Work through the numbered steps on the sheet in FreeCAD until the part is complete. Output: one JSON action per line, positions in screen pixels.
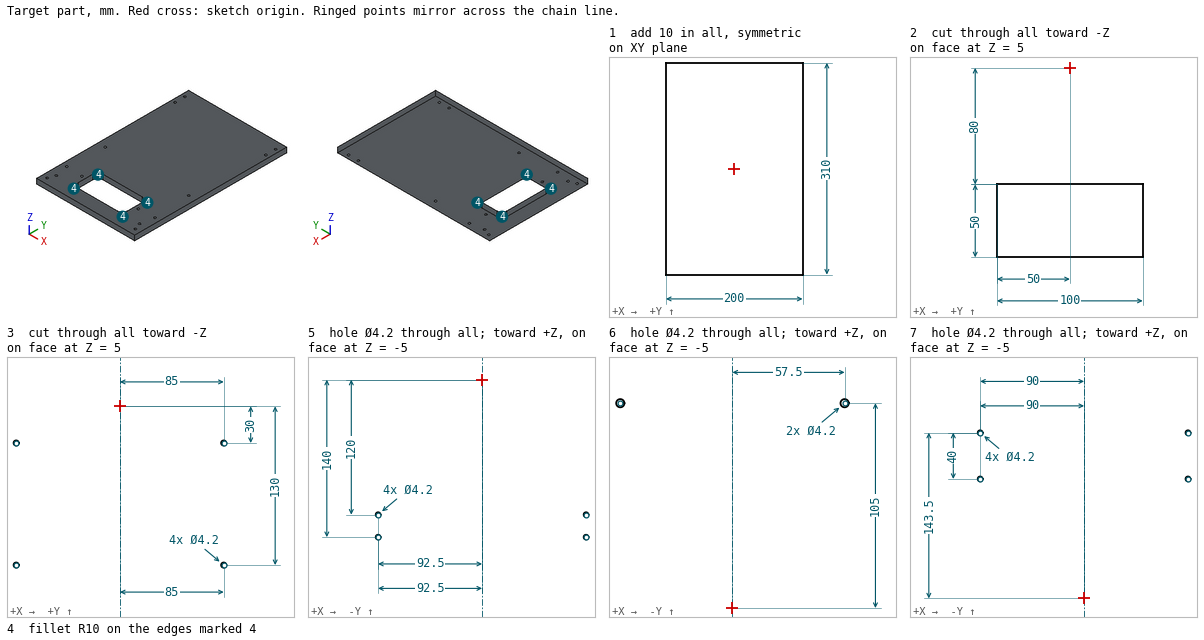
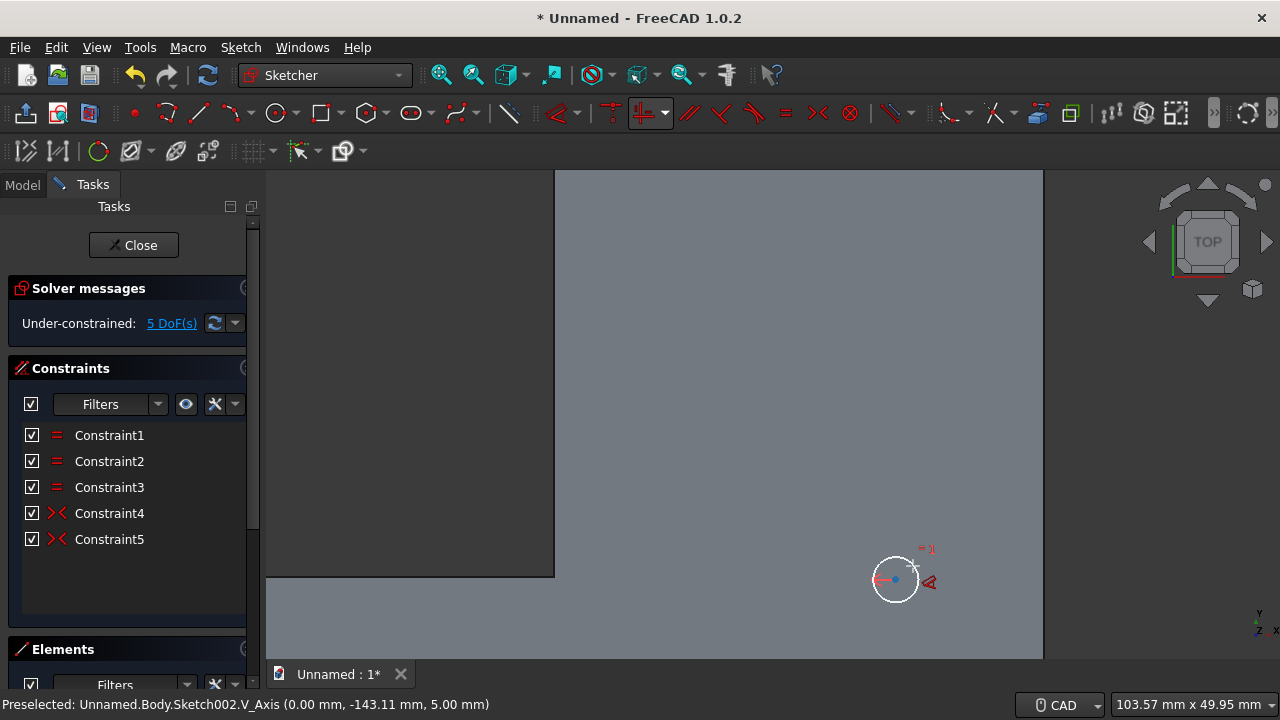
{"action": "left_click", "coordinate": [912, 564]}
{"action": "left_click", "coordinate": [935, 542]}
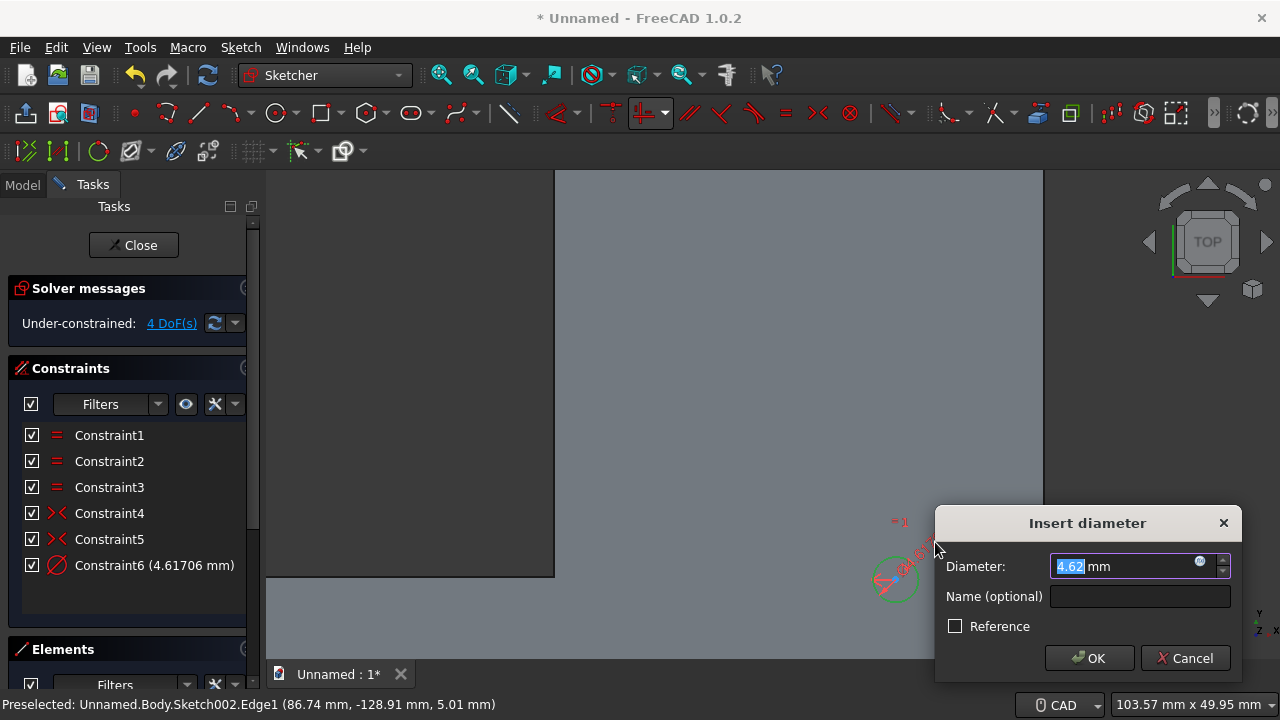
{"action": "type", "text": "4.2"}
{"action": "key", "text": "Return"}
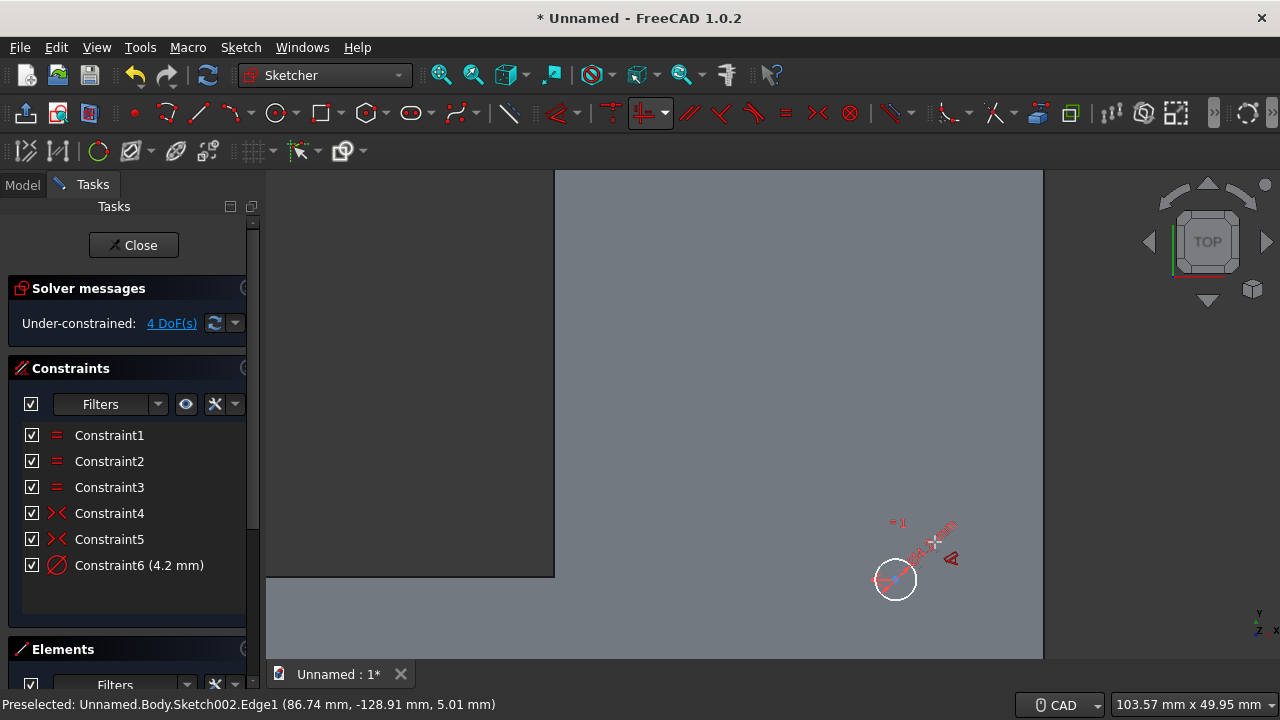
{"action": "scroll", "coordinate": [914, 566], "scroll_direction": "down", "scroll_amount": 7}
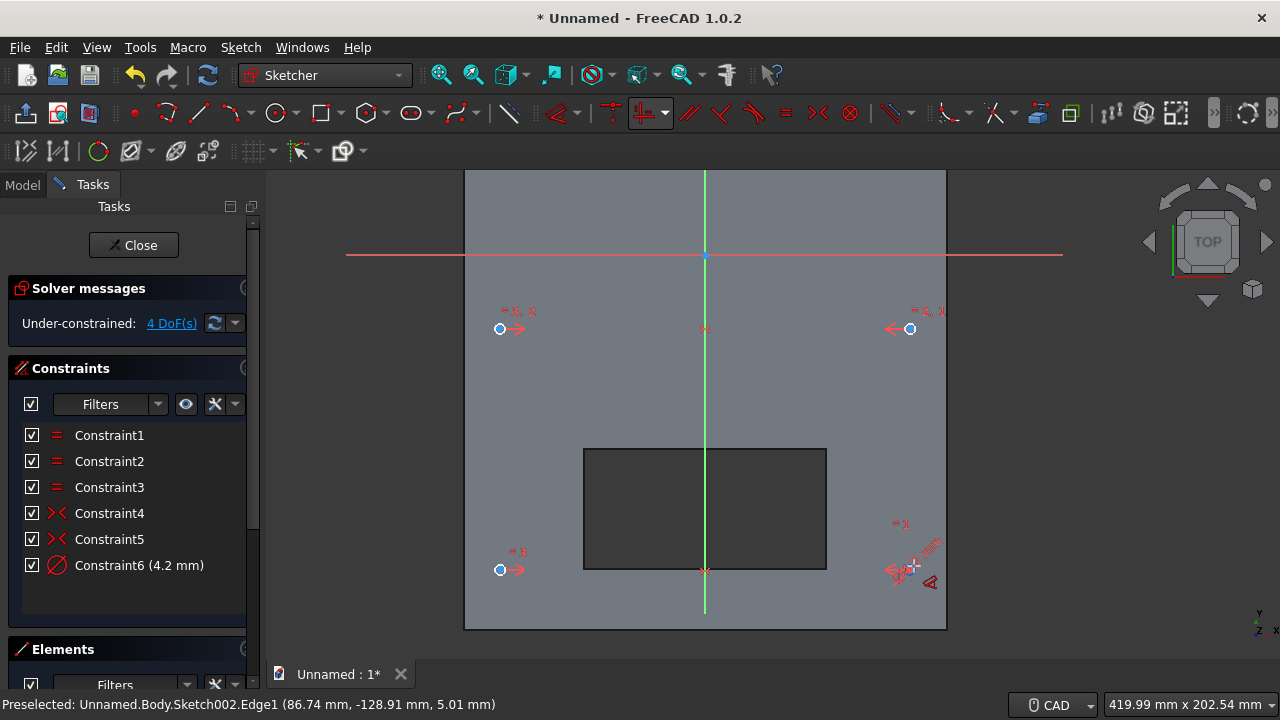
{"action": "left_click", "coordinate": [910, 570]}
{"action": "left_click", "coordinate": [808, 221]}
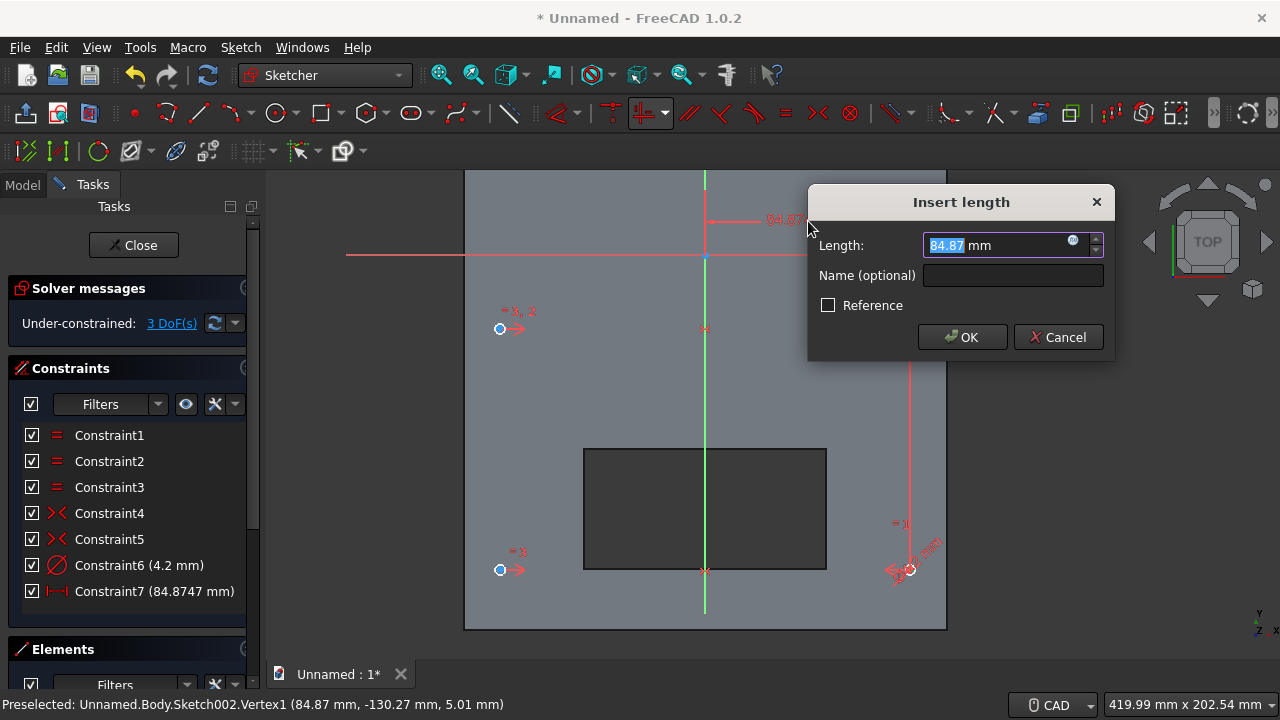
{"action": "type", "text": "85"}
{"action": "key", "text": "Return"}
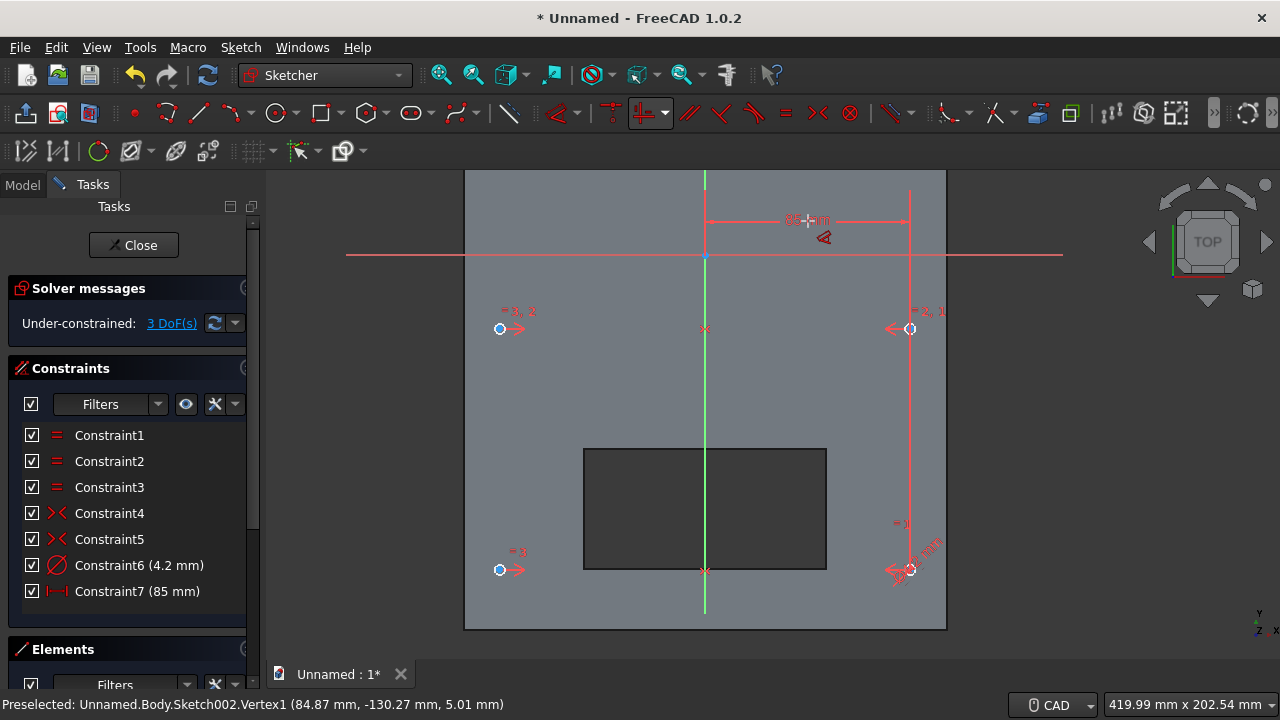
{"action": "left_click", "coordinate": [910, 329]}
{"action": "left_click", "coordinate": [736, 221]}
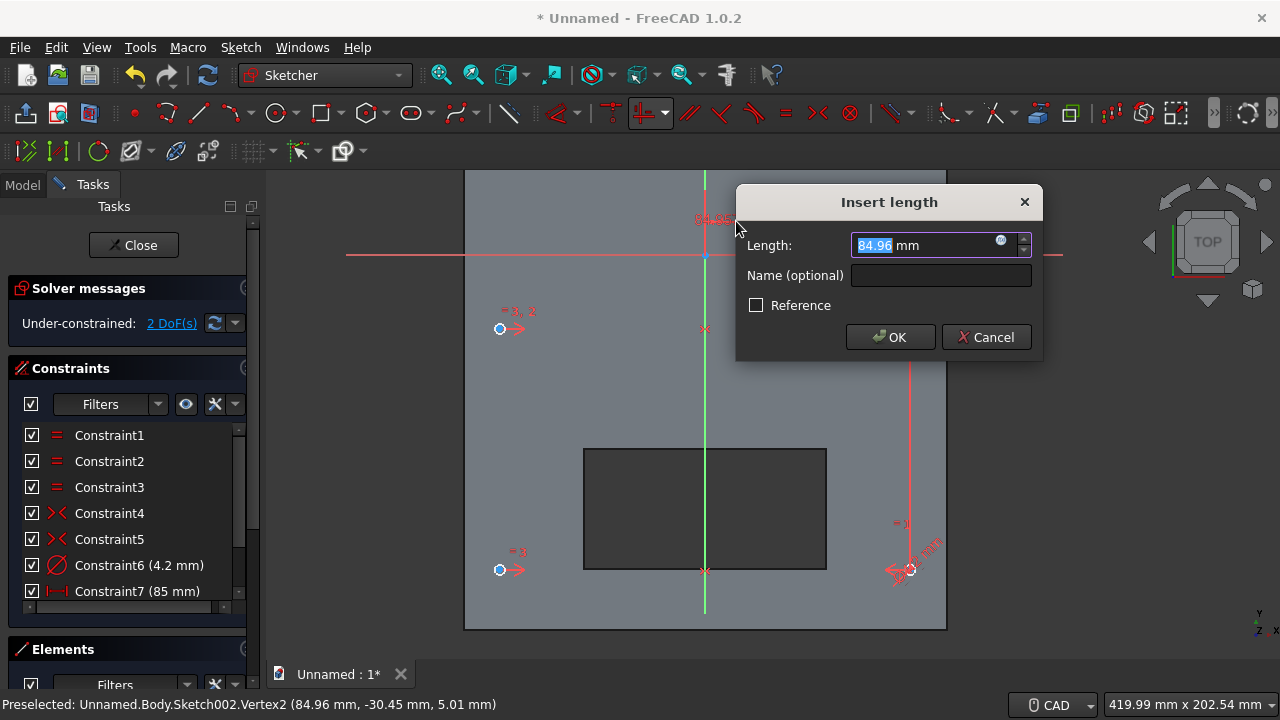
{"action": "type", "text": "85"}
{"action": "key", "text": "Return"}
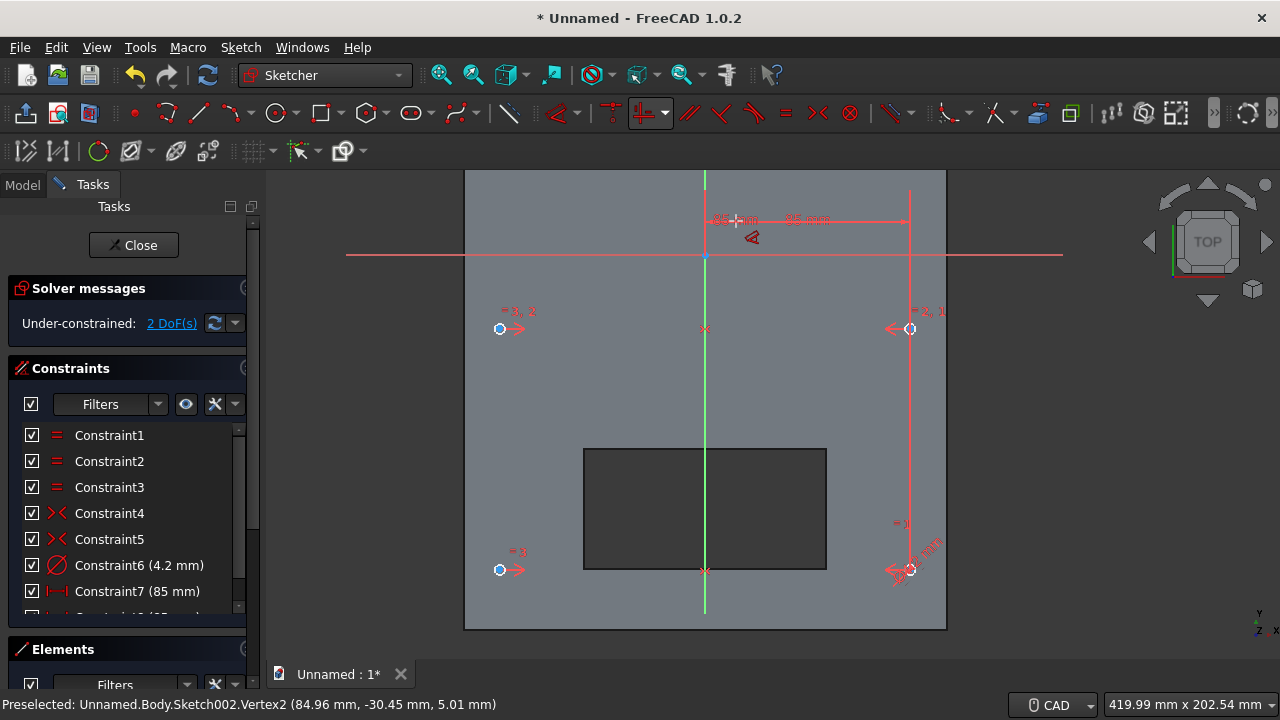
{"action": "left_click", "coordinate": [910, 329]}
{"action": "left_click", "coordinate": [944, 292]}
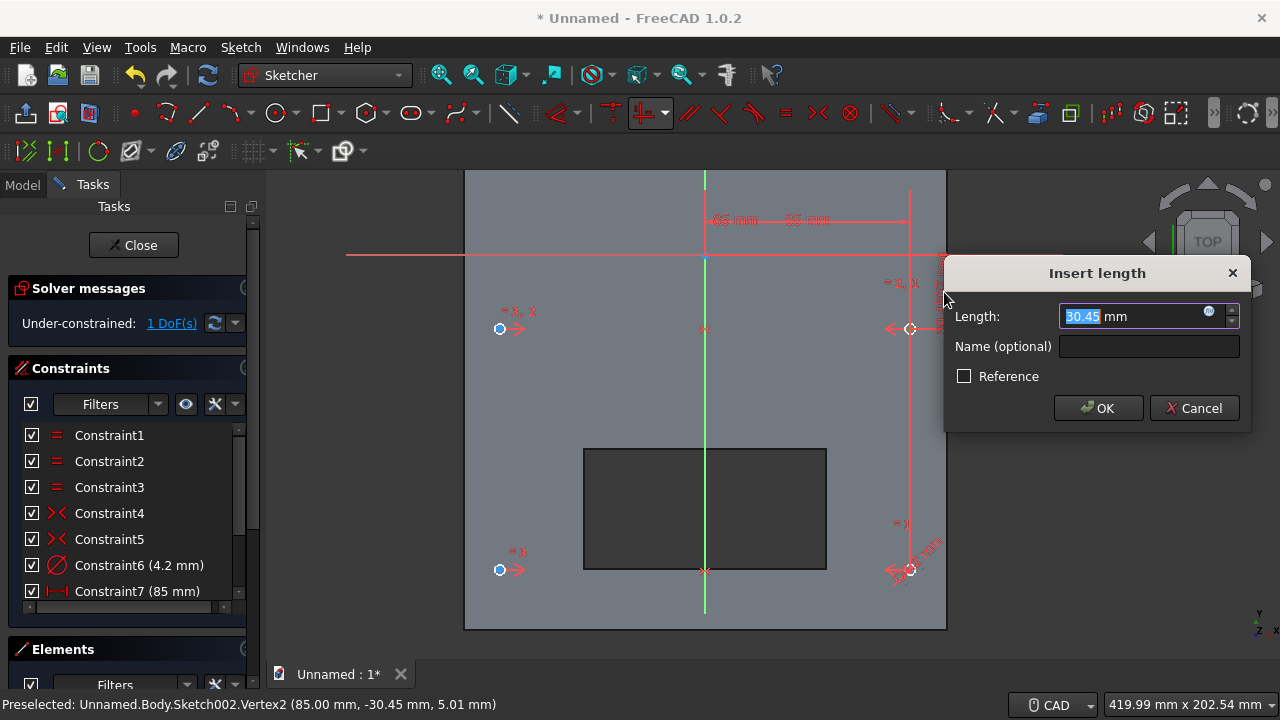
{"action": "type", "text": "30"}
{"action": "key", "text": "Return"}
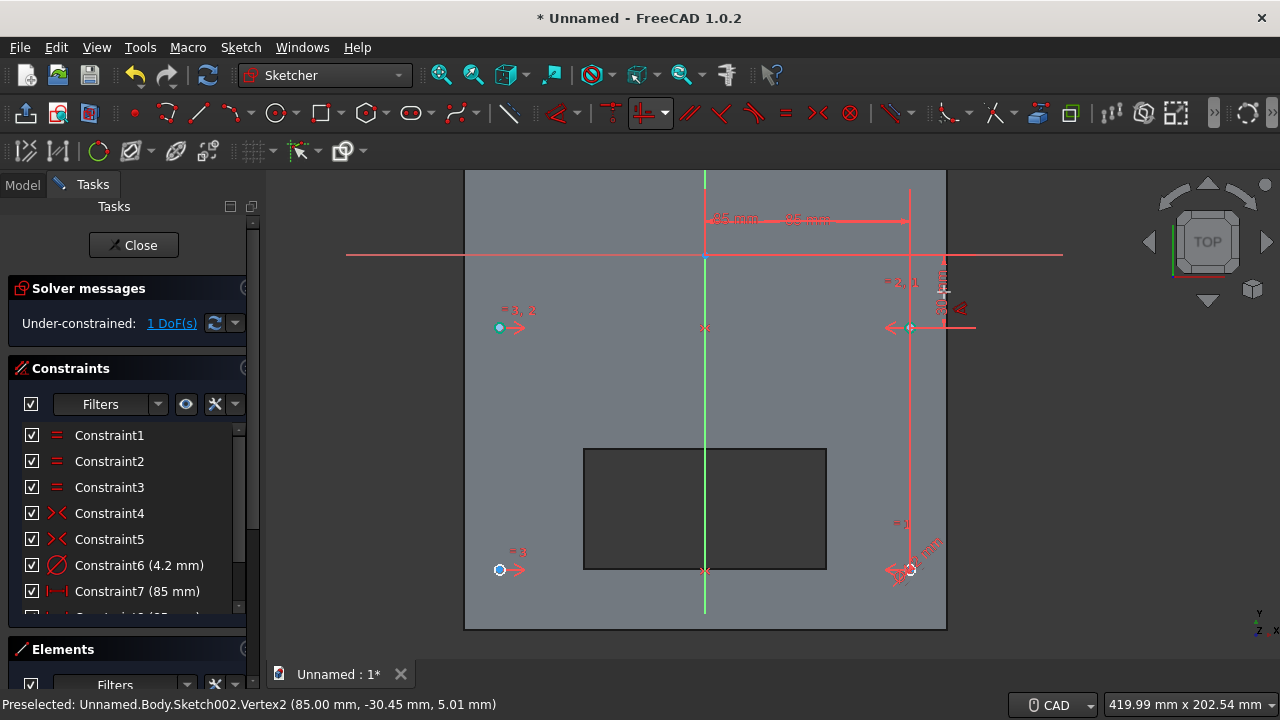
{"action": "left_click", "coordinate": [910, 570]}
{"action": "left_click", "coordinate": [944, 413]}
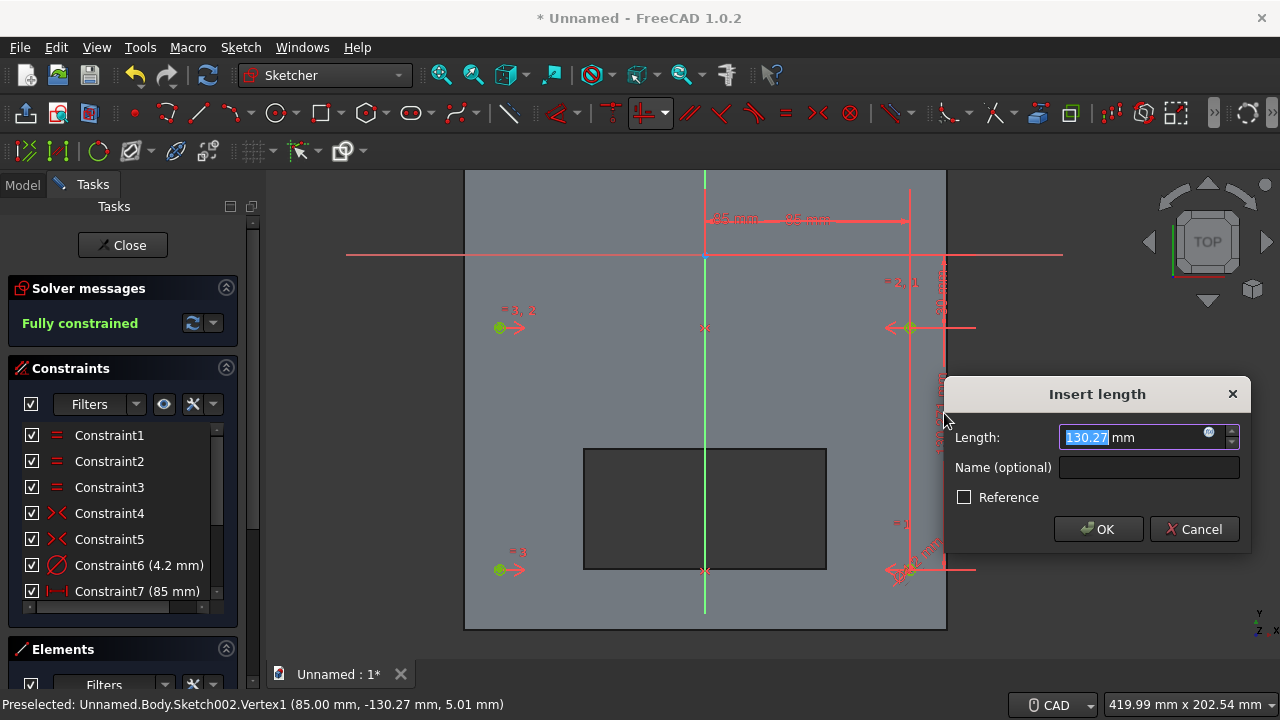
{"action": "type", "text": "130"}
{"action": "key", "text": "Return"}
{"action": "key", "text": "Escape"}